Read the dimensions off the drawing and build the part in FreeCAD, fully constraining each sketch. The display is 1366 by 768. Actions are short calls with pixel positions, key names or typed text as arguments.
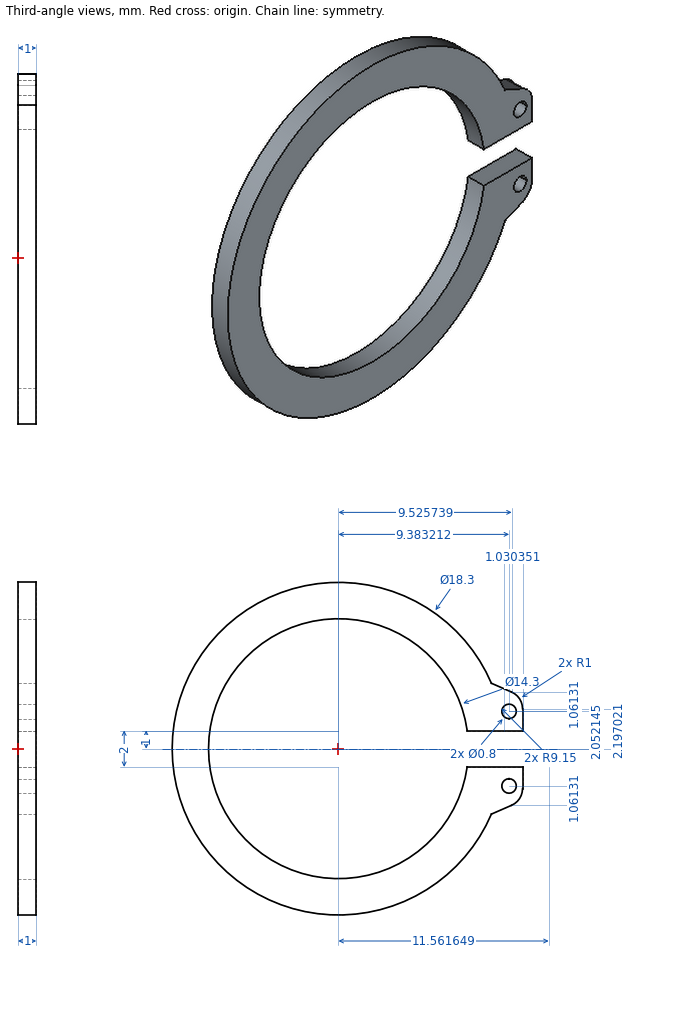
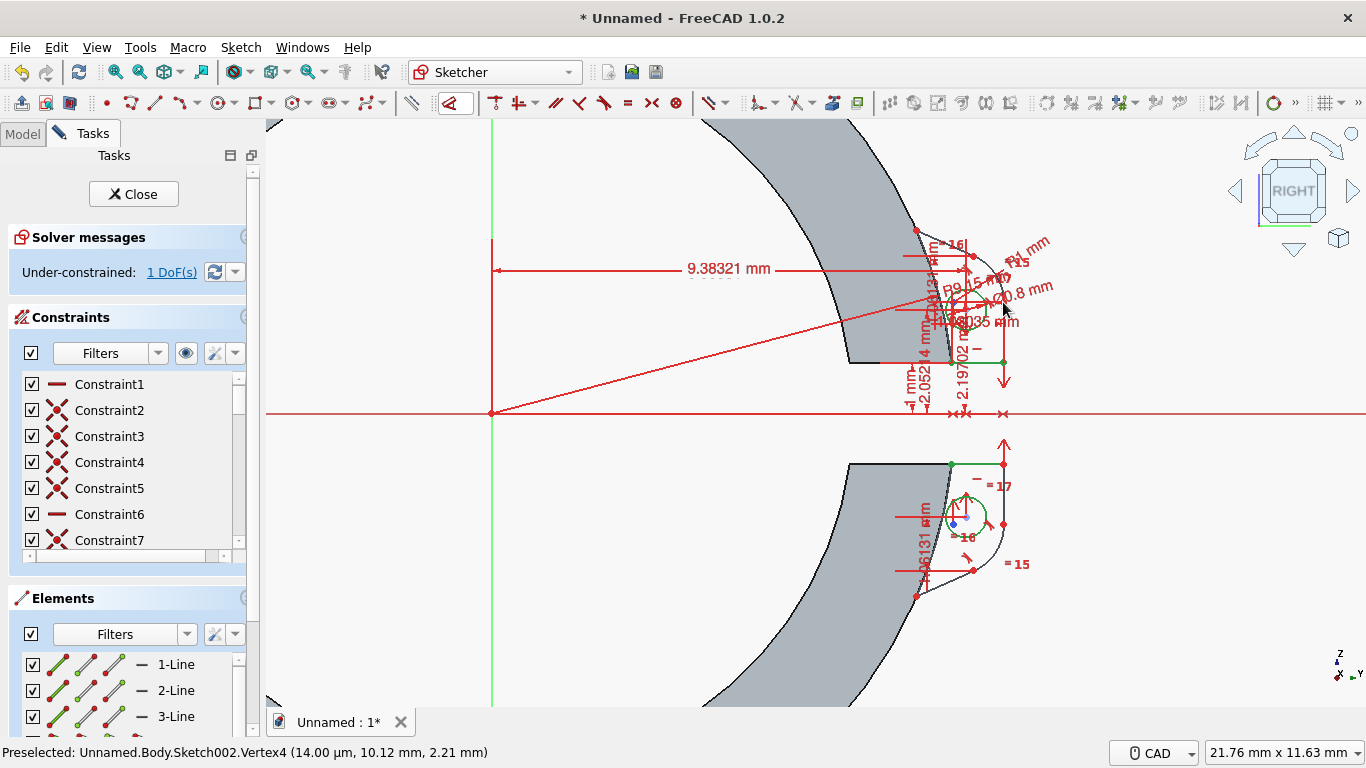
click(974, 256)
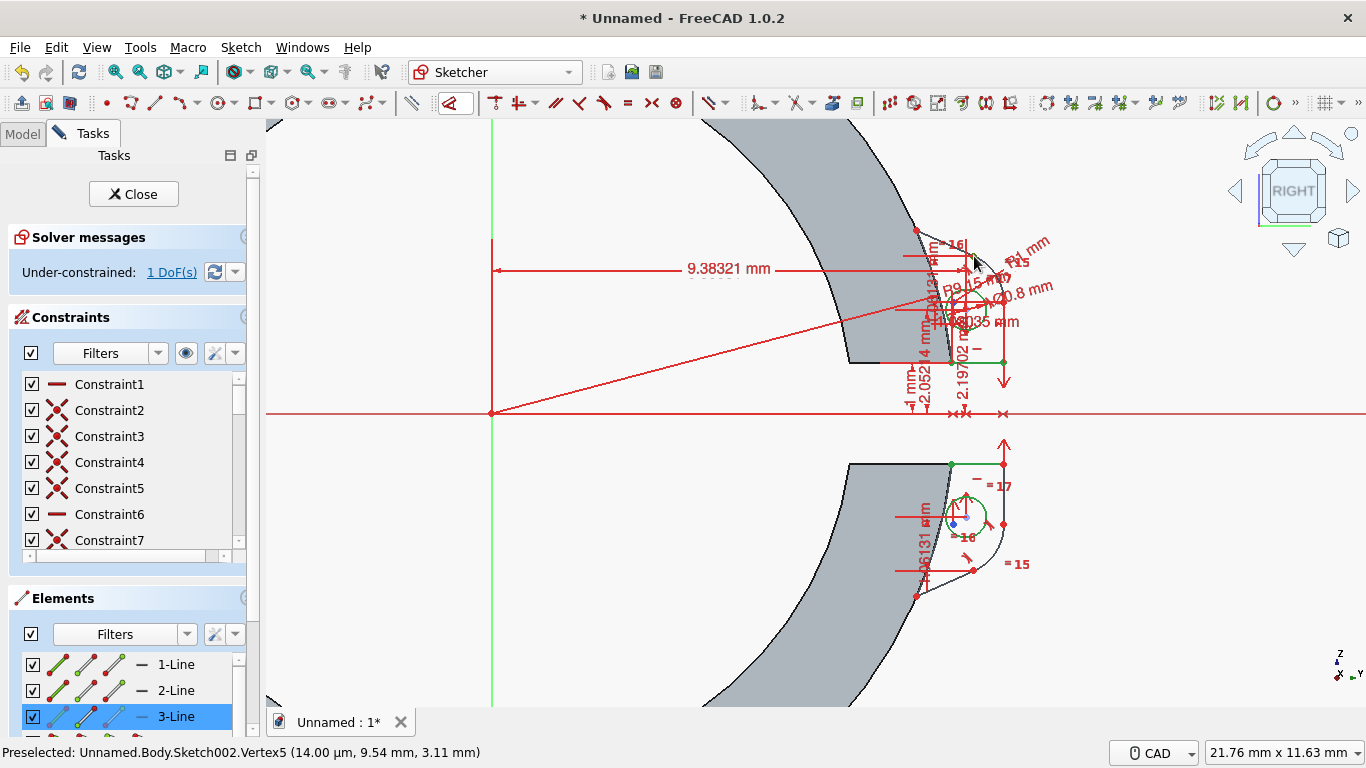
click(468, 104)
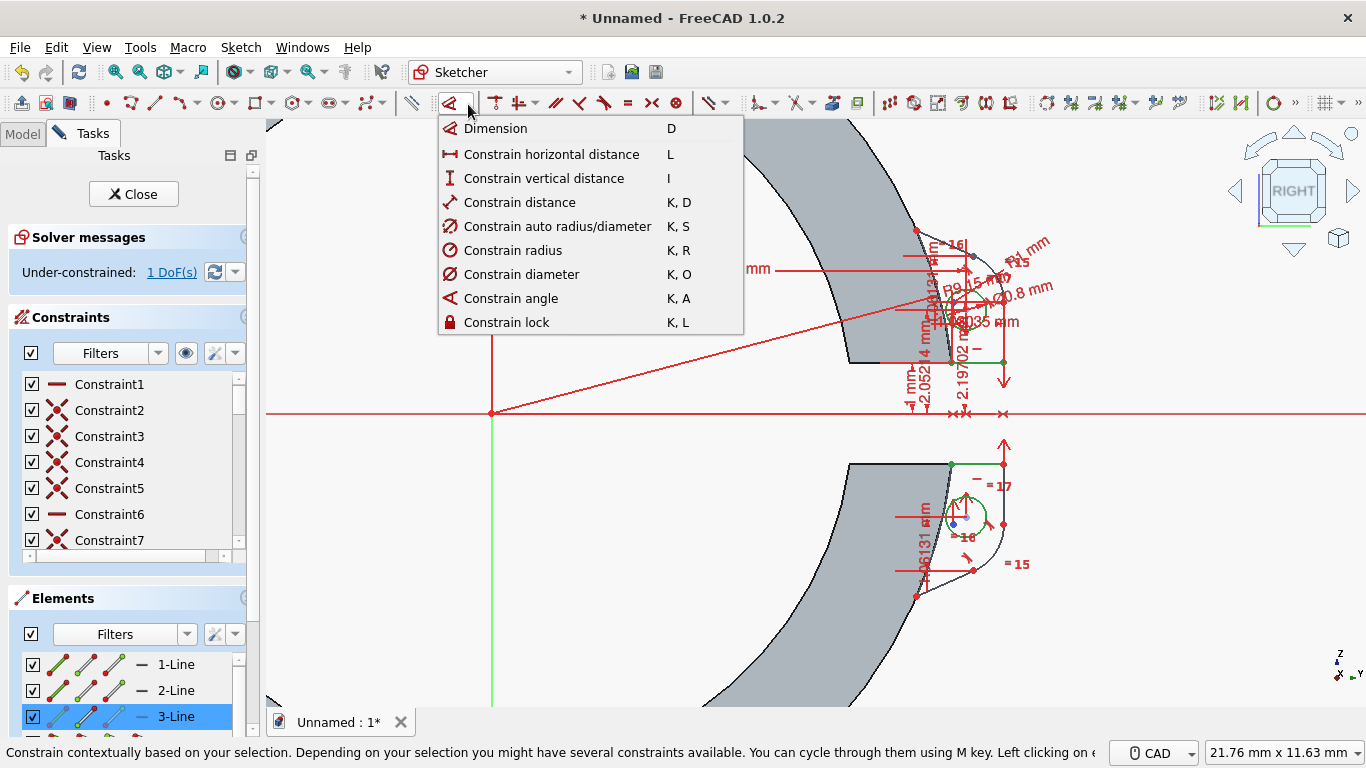
click(591, 154)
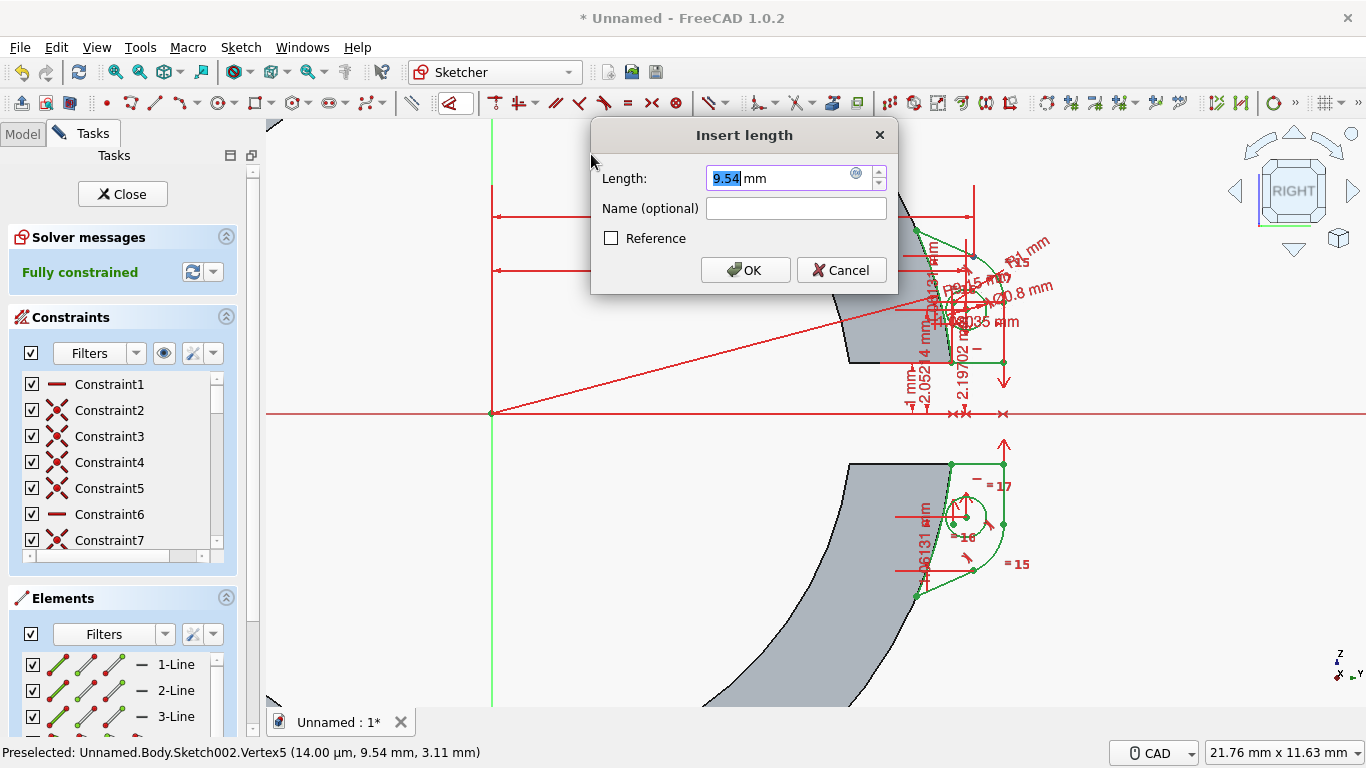
text(9.525739)
key(Return)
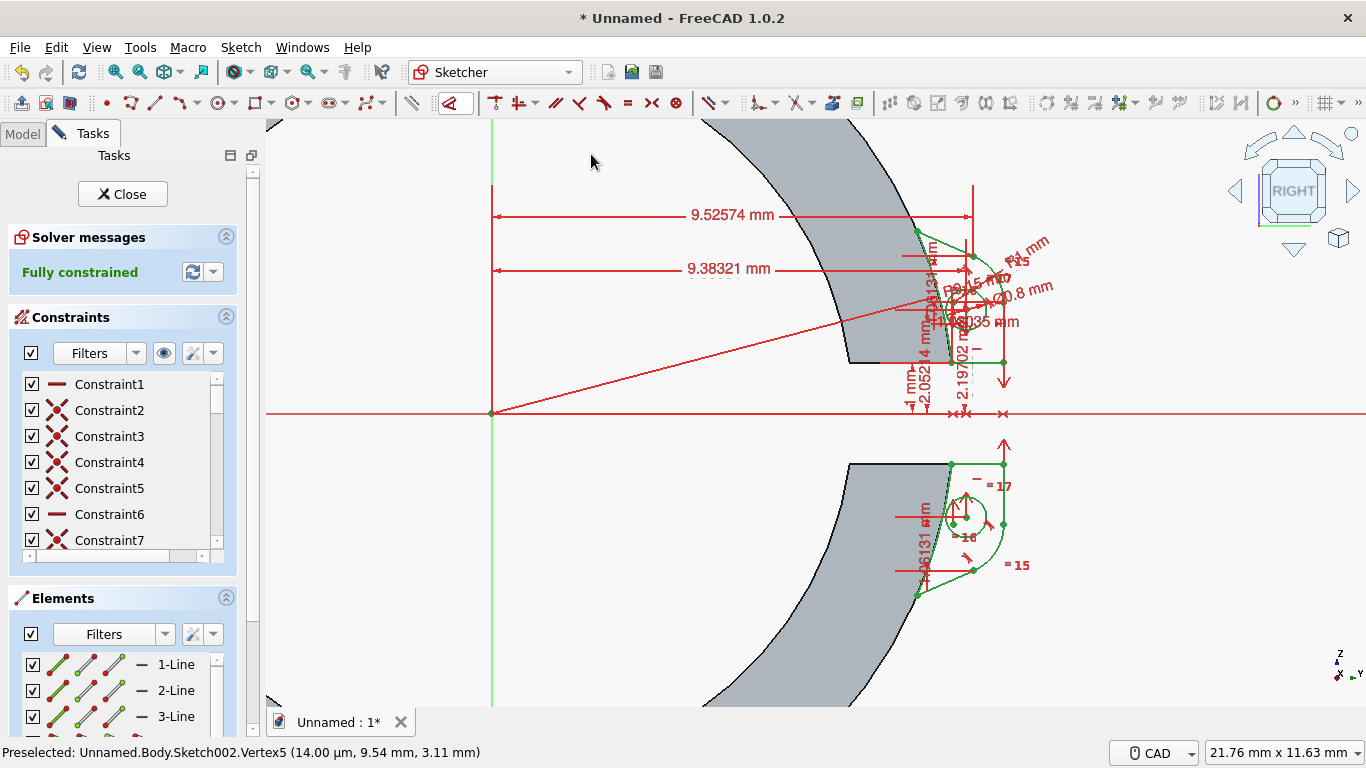
click(123, 194)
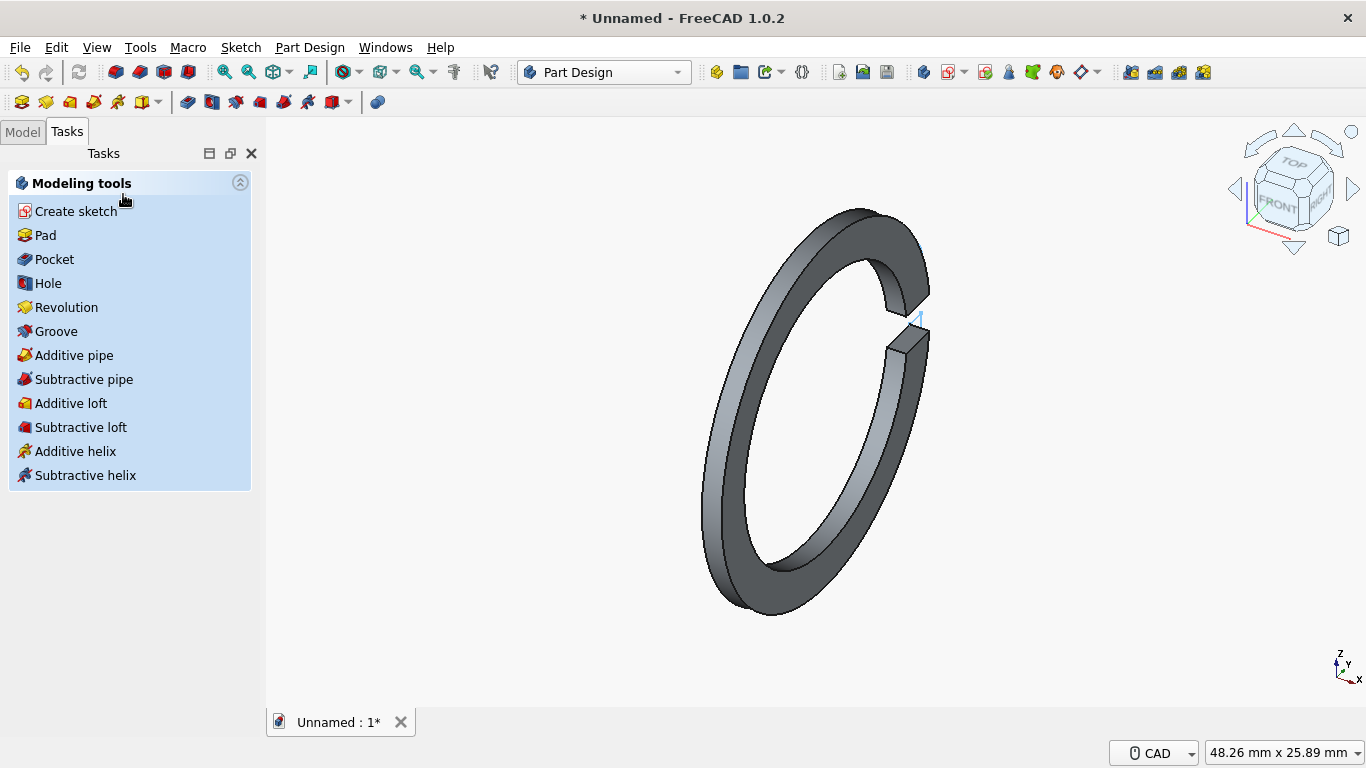
click(22, 102)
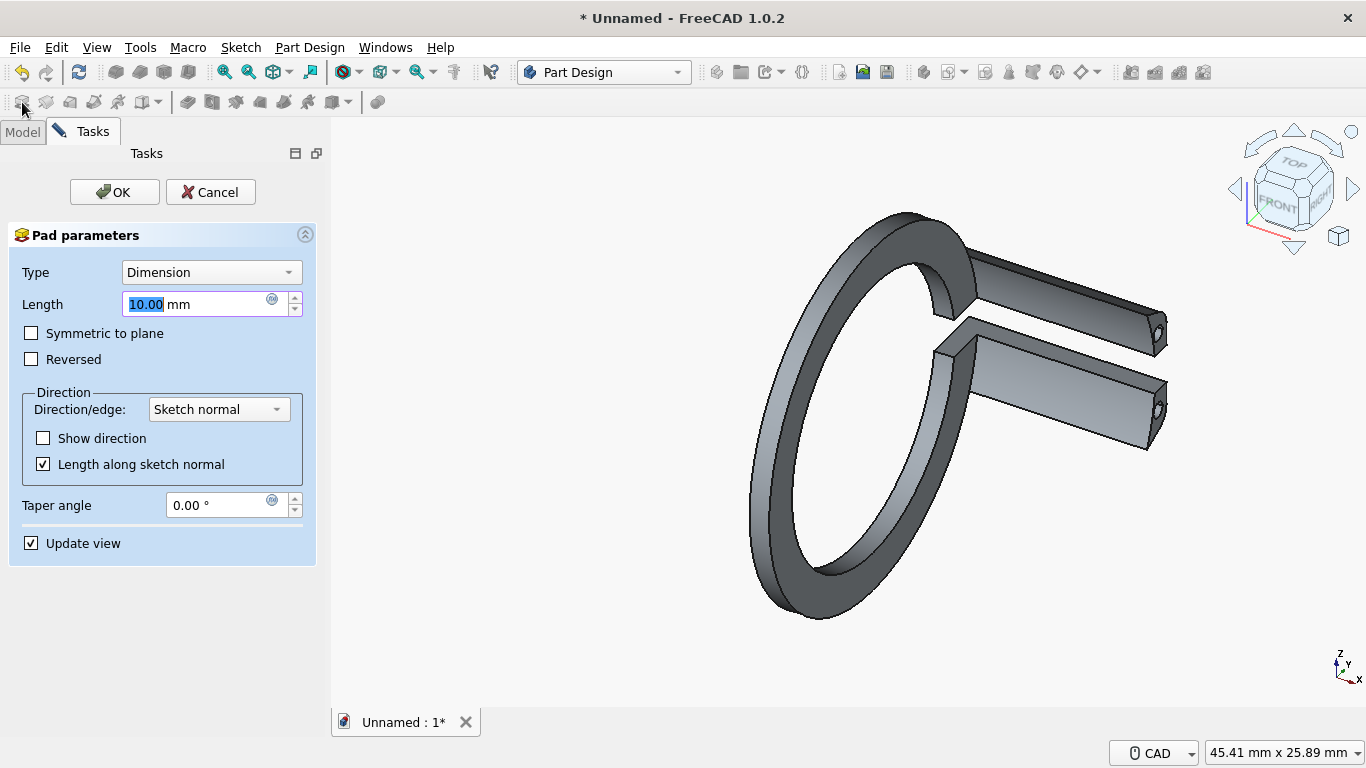
text(1)
key(Tab)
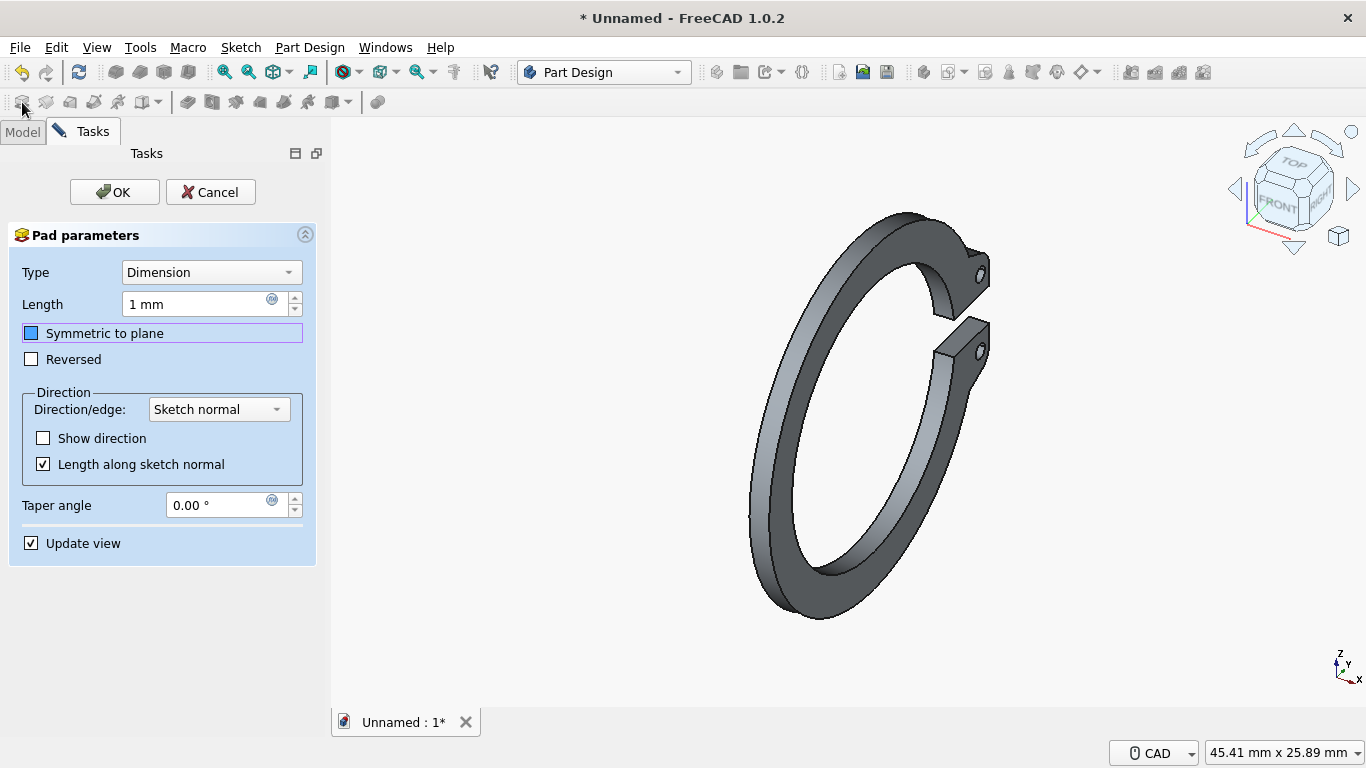
click(115, 192)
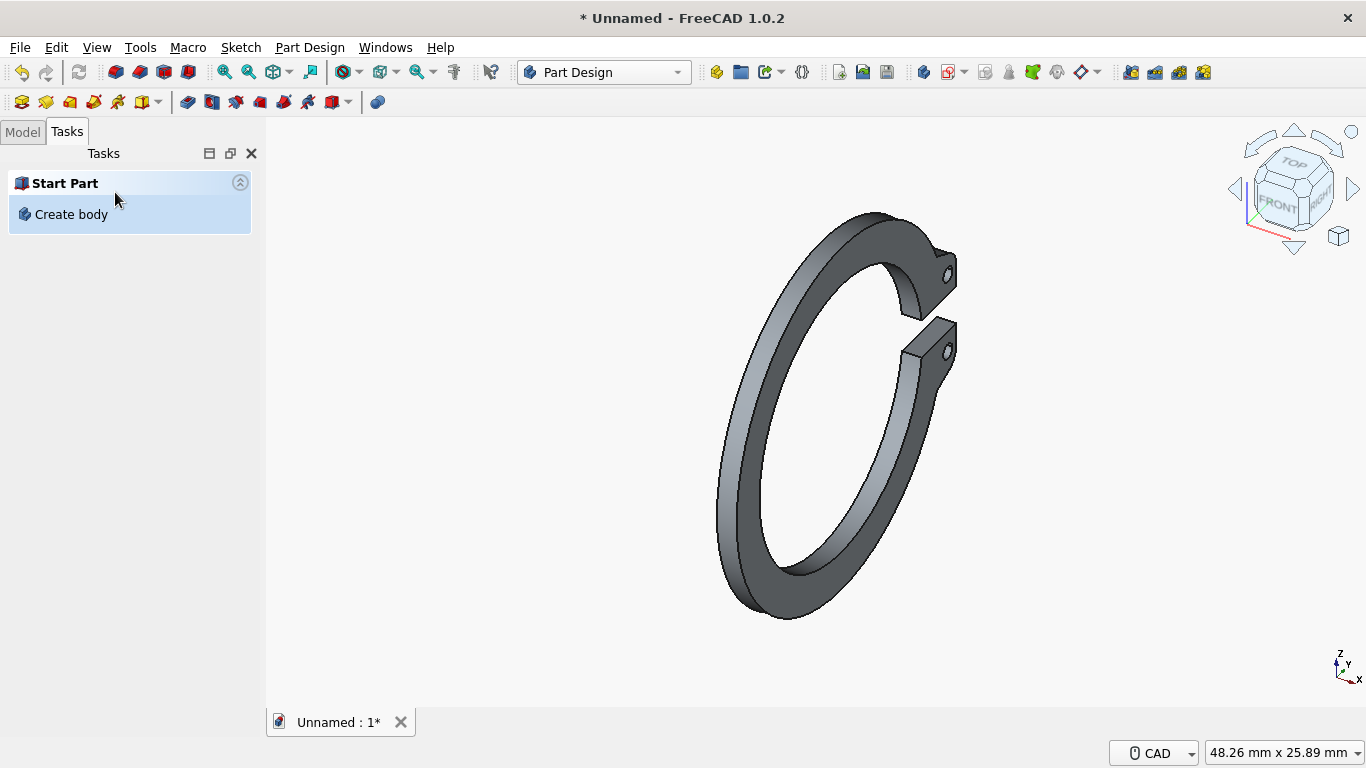
key(0)